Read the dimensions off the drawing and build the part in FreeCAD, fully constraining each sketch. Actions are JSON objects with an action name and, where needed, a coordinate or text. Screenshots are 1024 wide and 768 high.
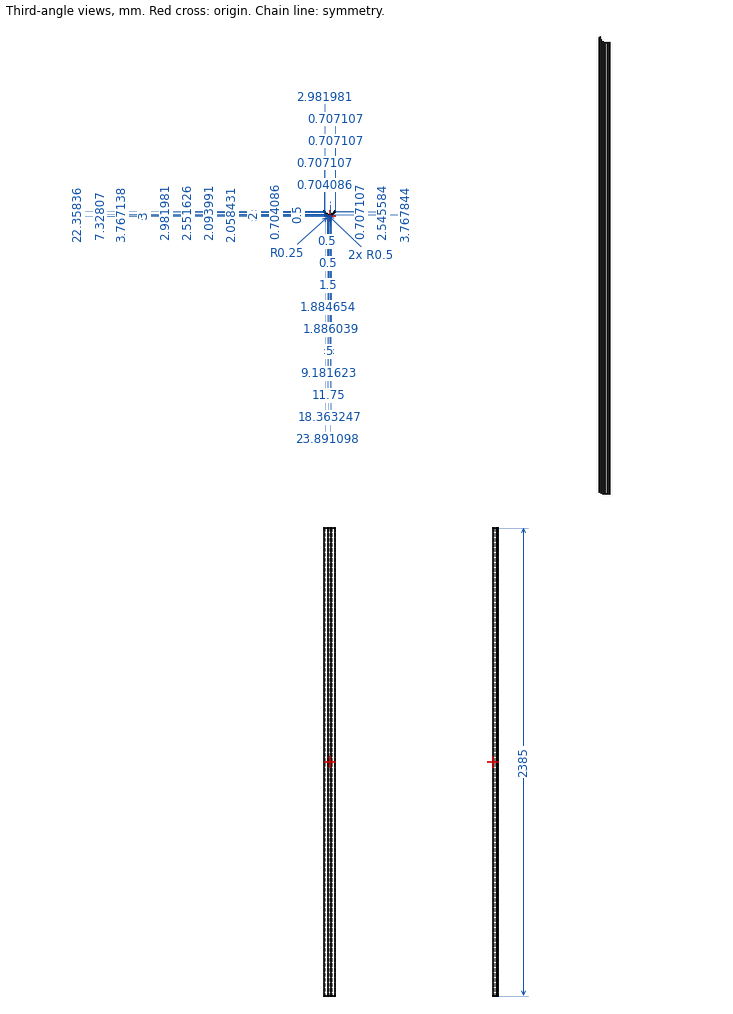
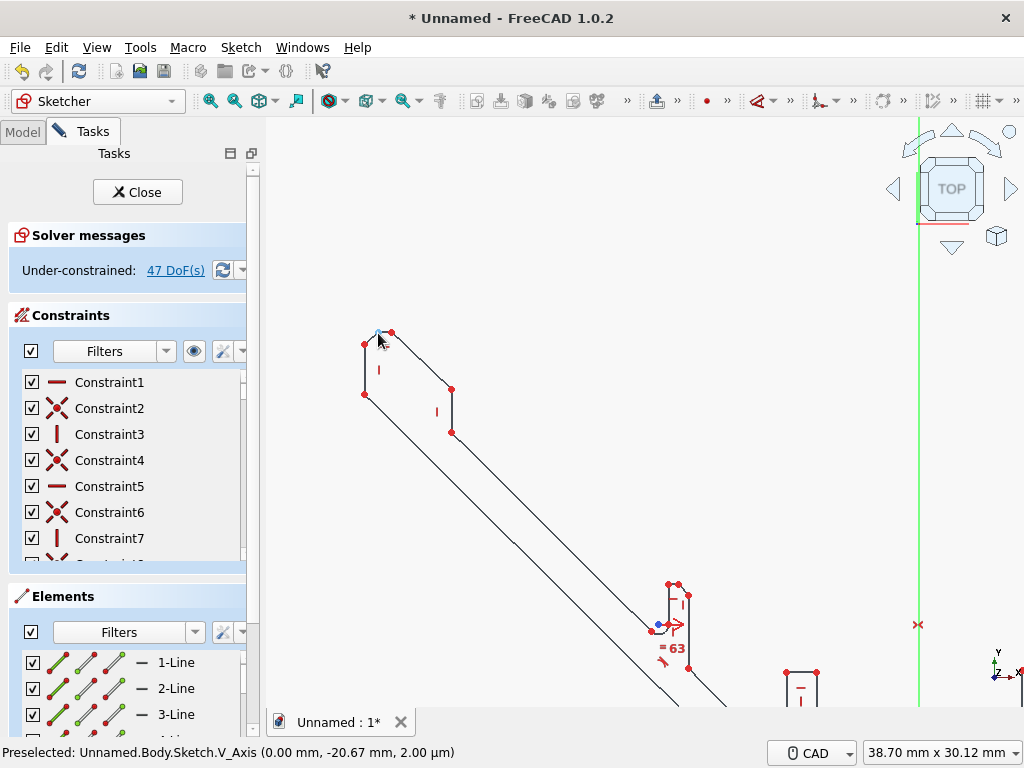
{"action": "left_click", "coordinate": [379, 332]}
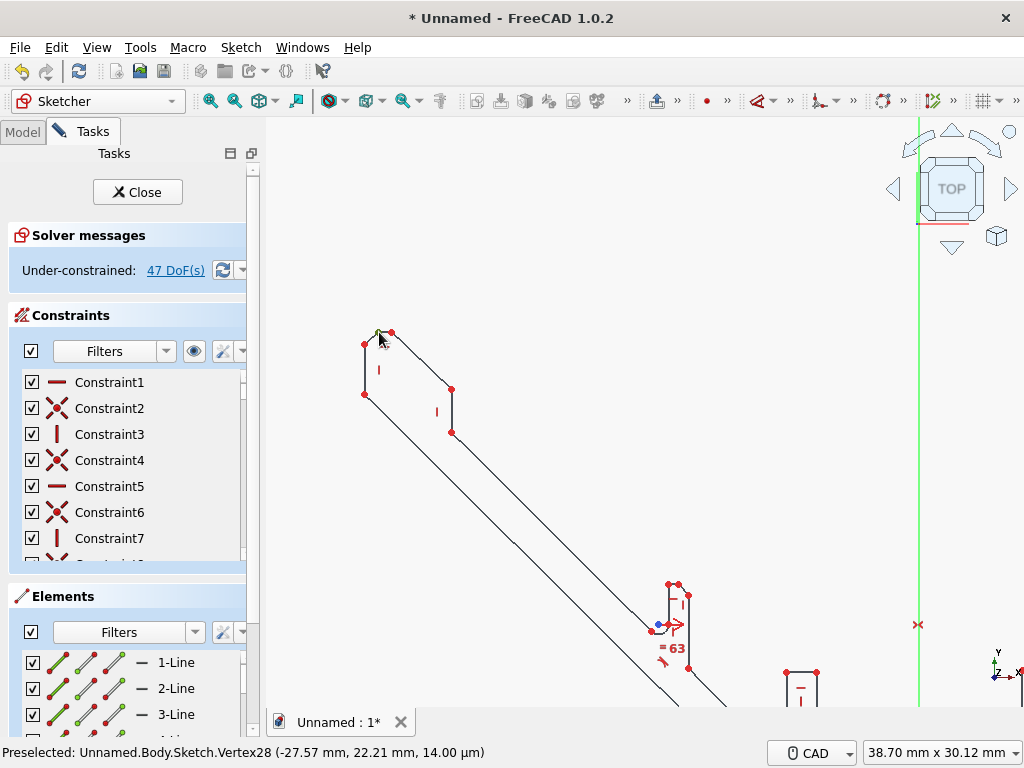
{"action": "scroll", "coordinate": [377, 333], "scroll_direction": "down", "scroll_amount": 5}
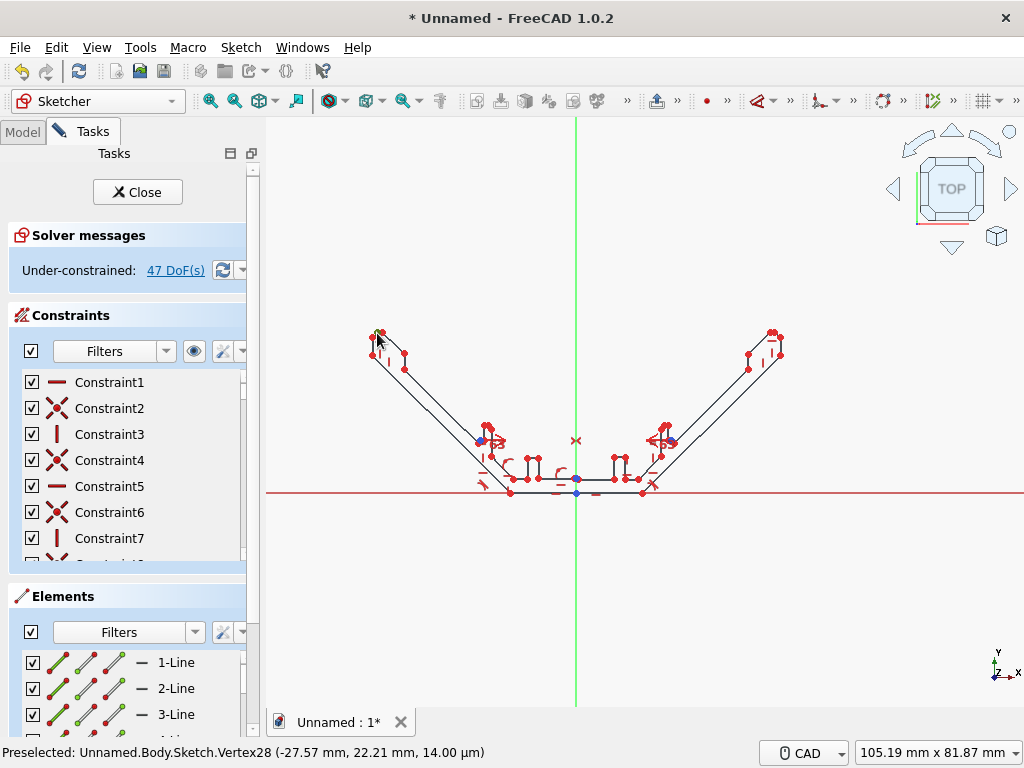
{"action": "scroll", "coordinate": [775, 332], "scroll_direction": "up", "scroll_amount": 5}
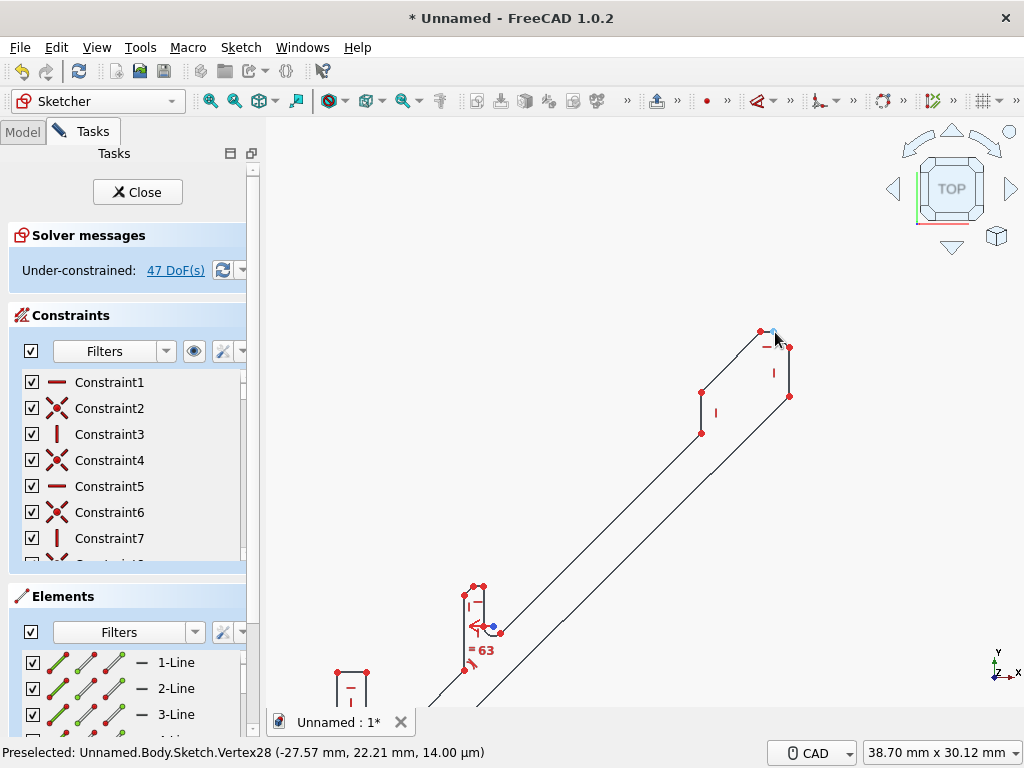
{"action": "left_click", "coordinate": [774, 332]}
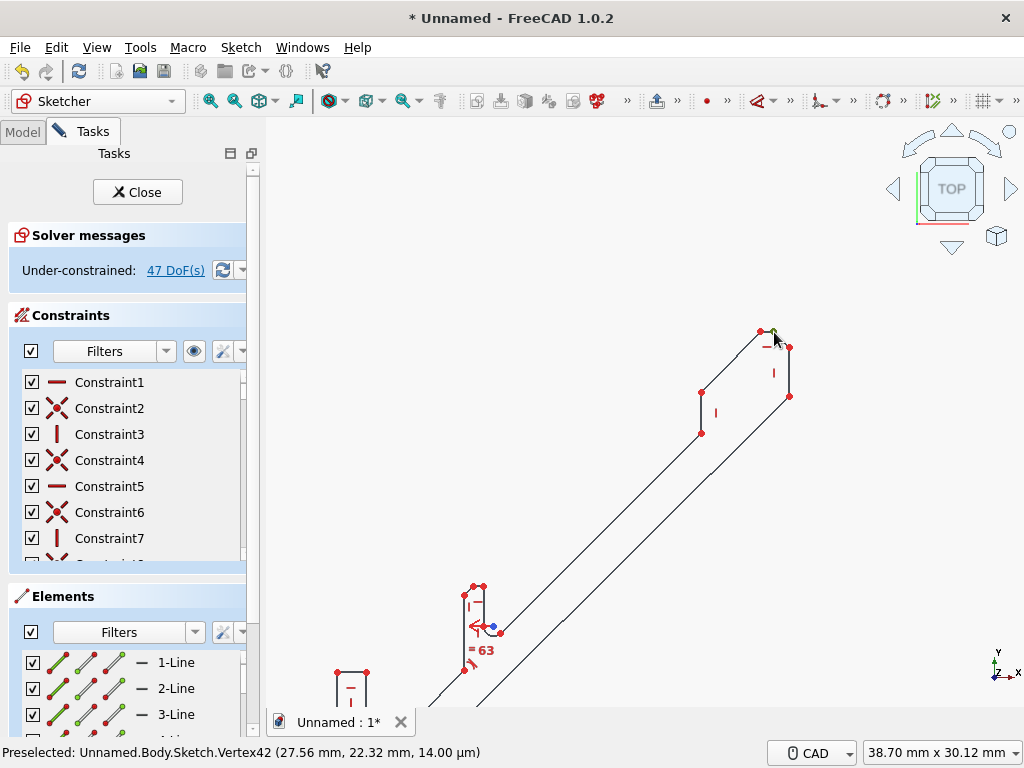
{"action": "scroll", "coordinate": [776, 332], "scroll_direction": "down", "scroll_amount": 5}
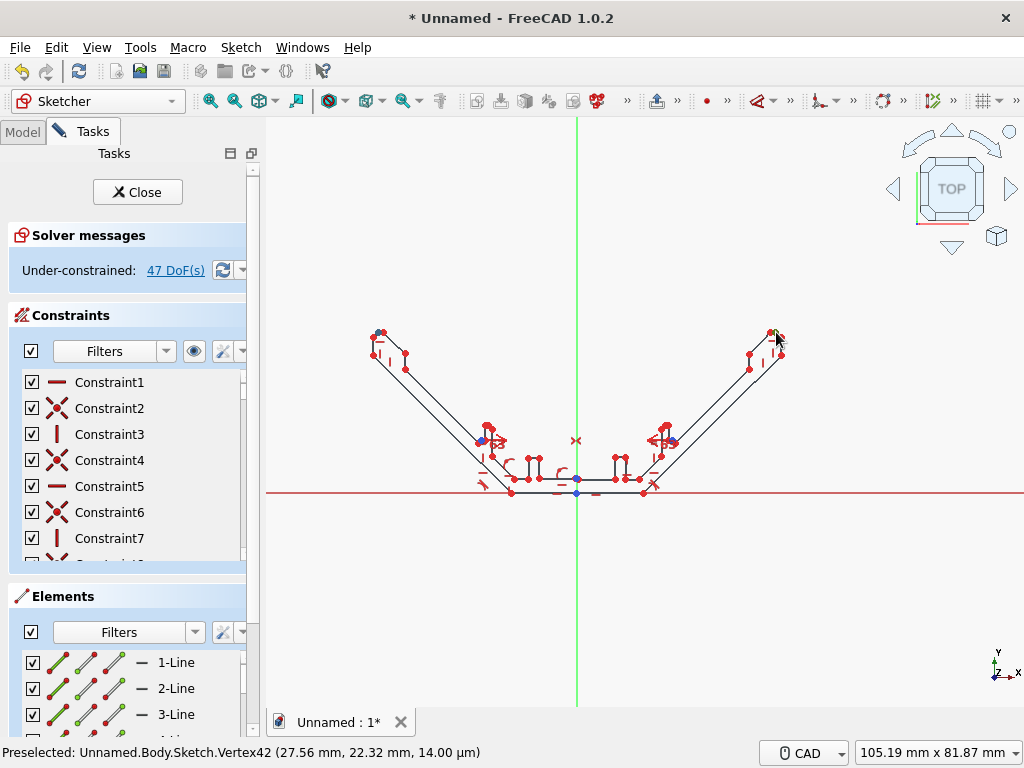
{"action": "left_click", "coordinate": [577, 641]}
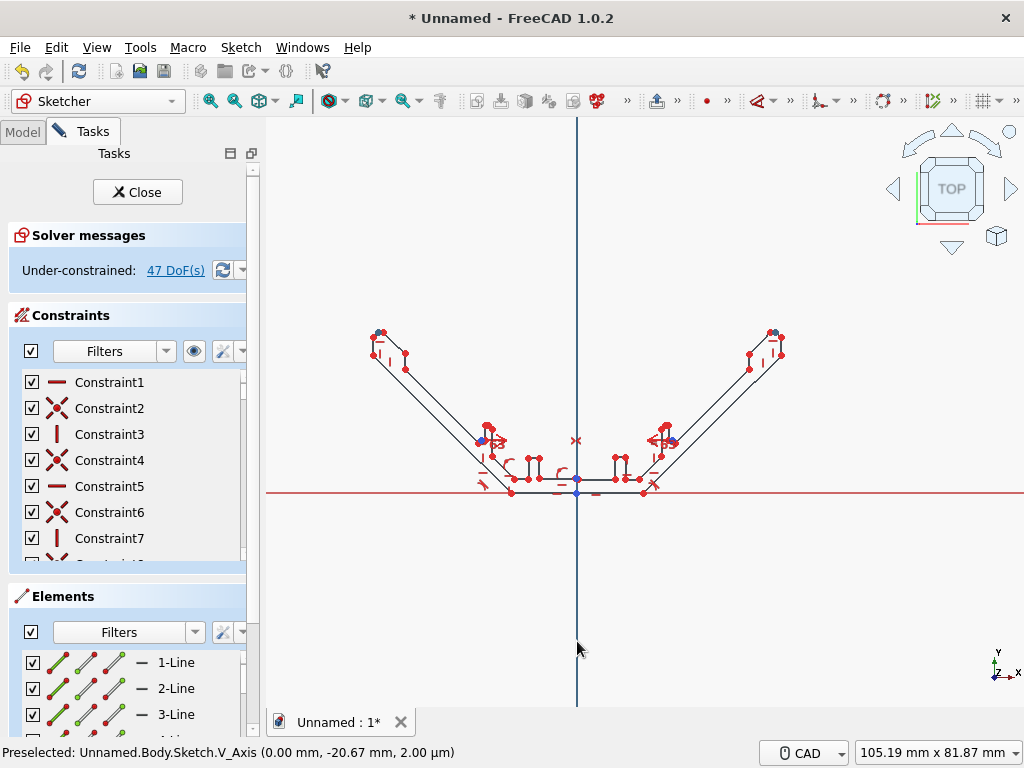
{"action": "key", "text": "s"}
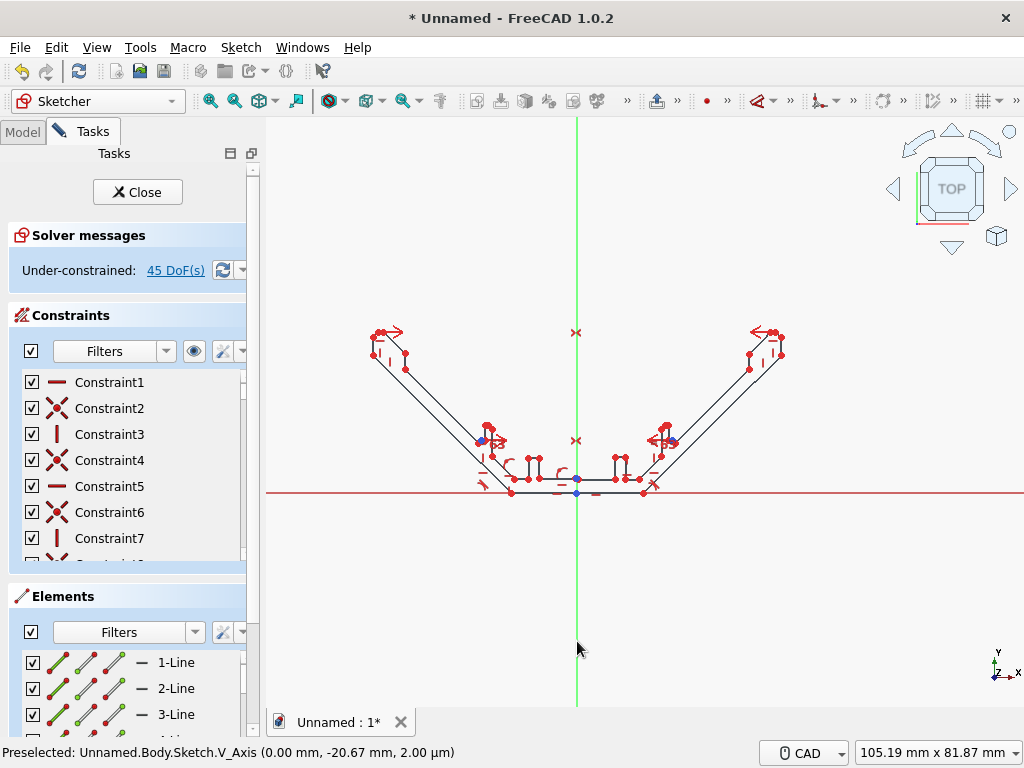
{"action": "left_click", "coordinate": [405, 354]}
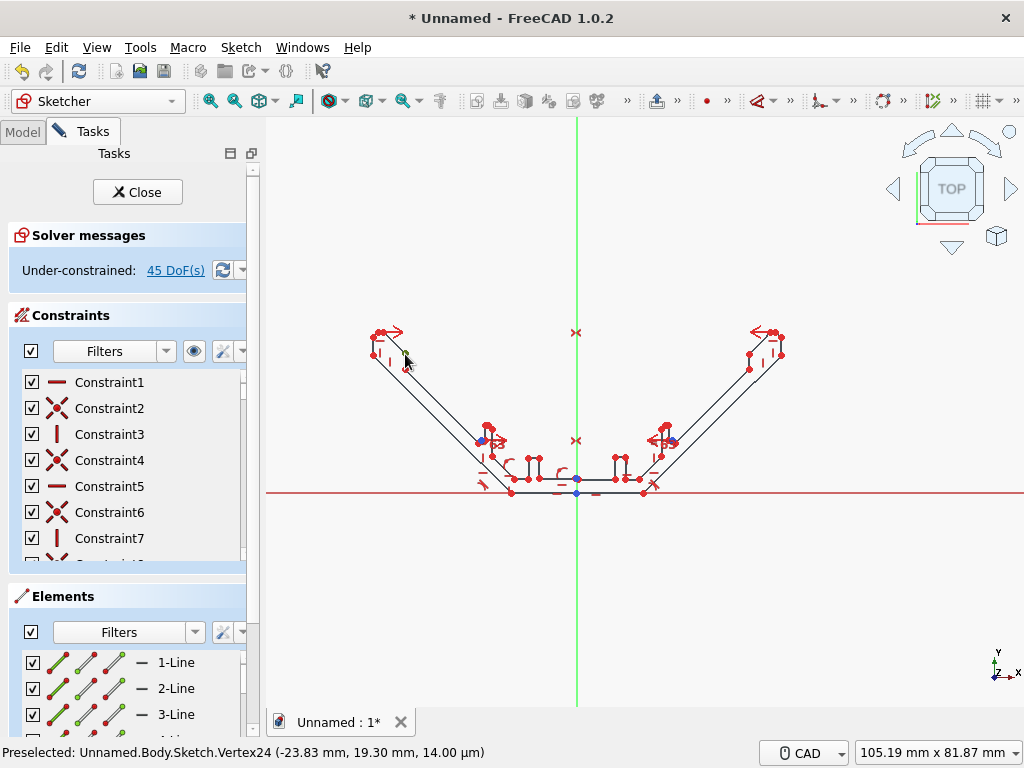
{"action": "left_click", "coordinate": [749, 355]}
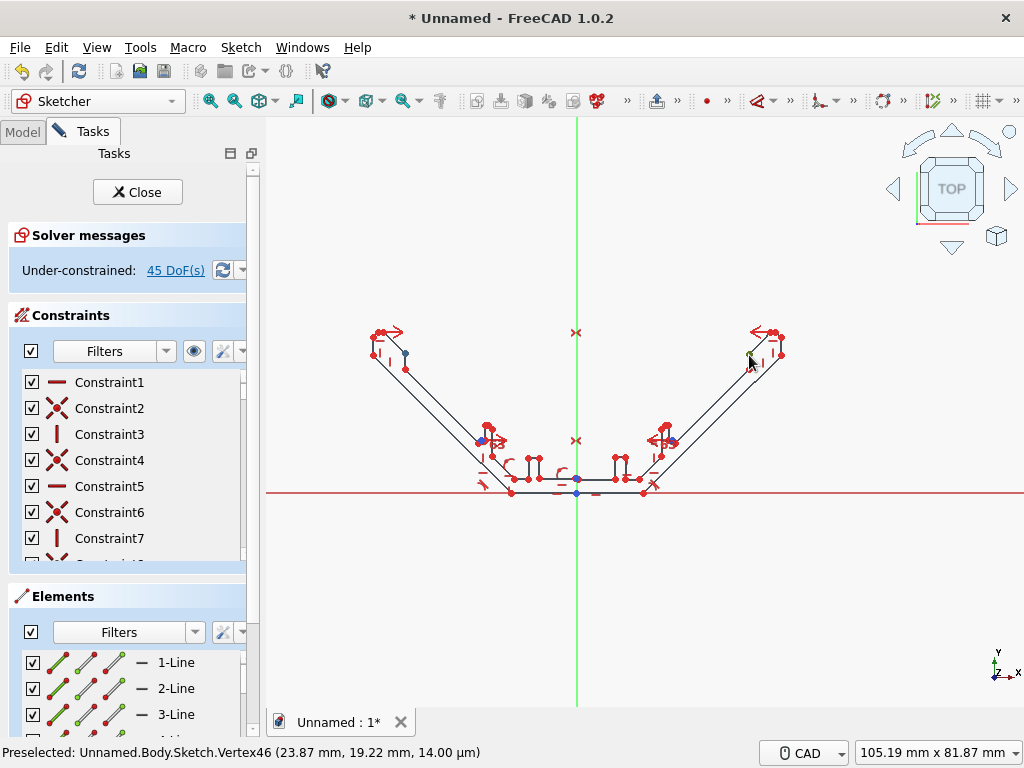
{"action": "left_click", "coordinate": [577, 641]}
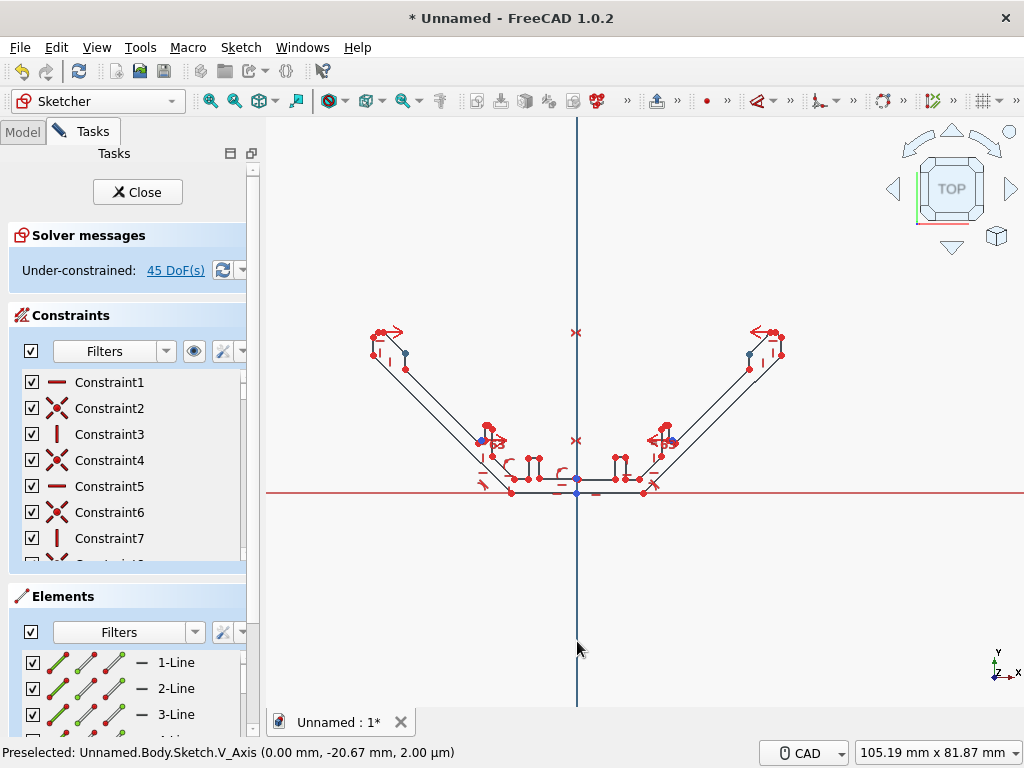
{"action": "key", "text": "s"}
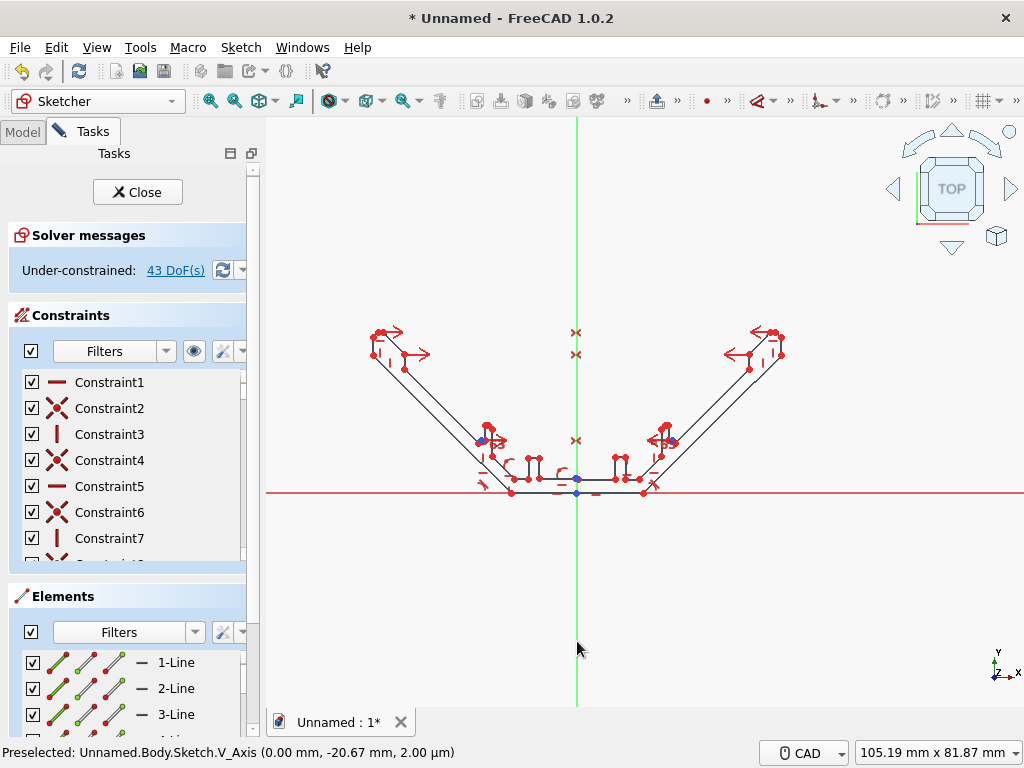
{"action": "scroll", "coordinate": [489, 426], "scroll_direction": "up", "scroll_amount": 6}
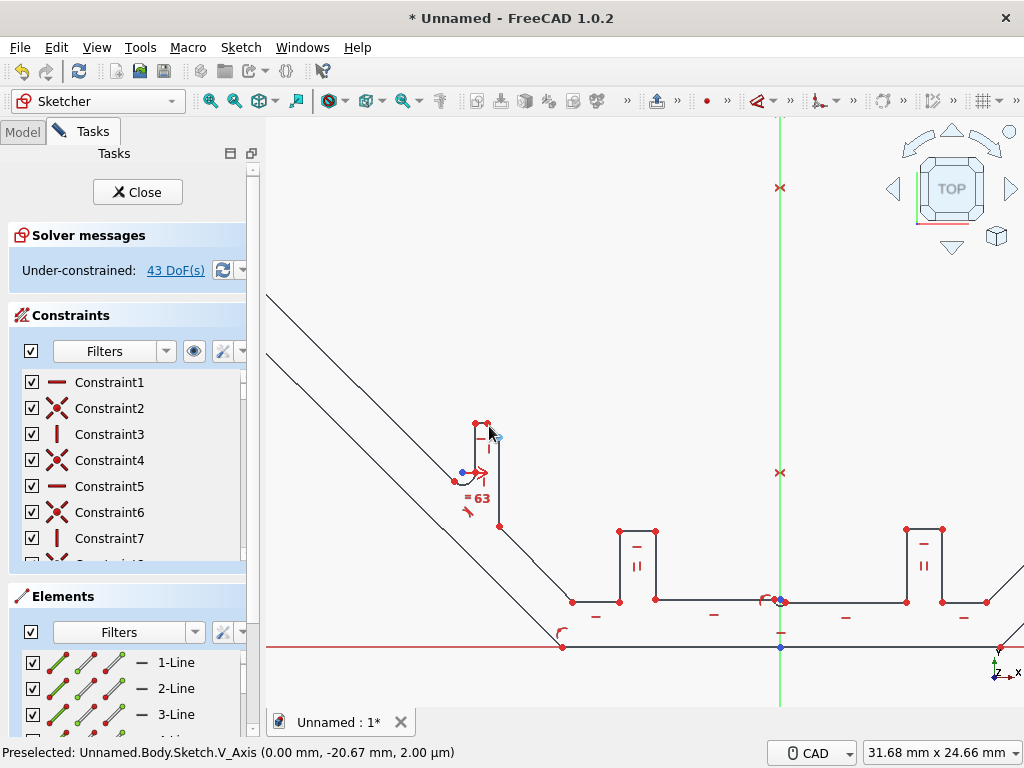
{"action": "left_click", "coordinate": [488, 423]}